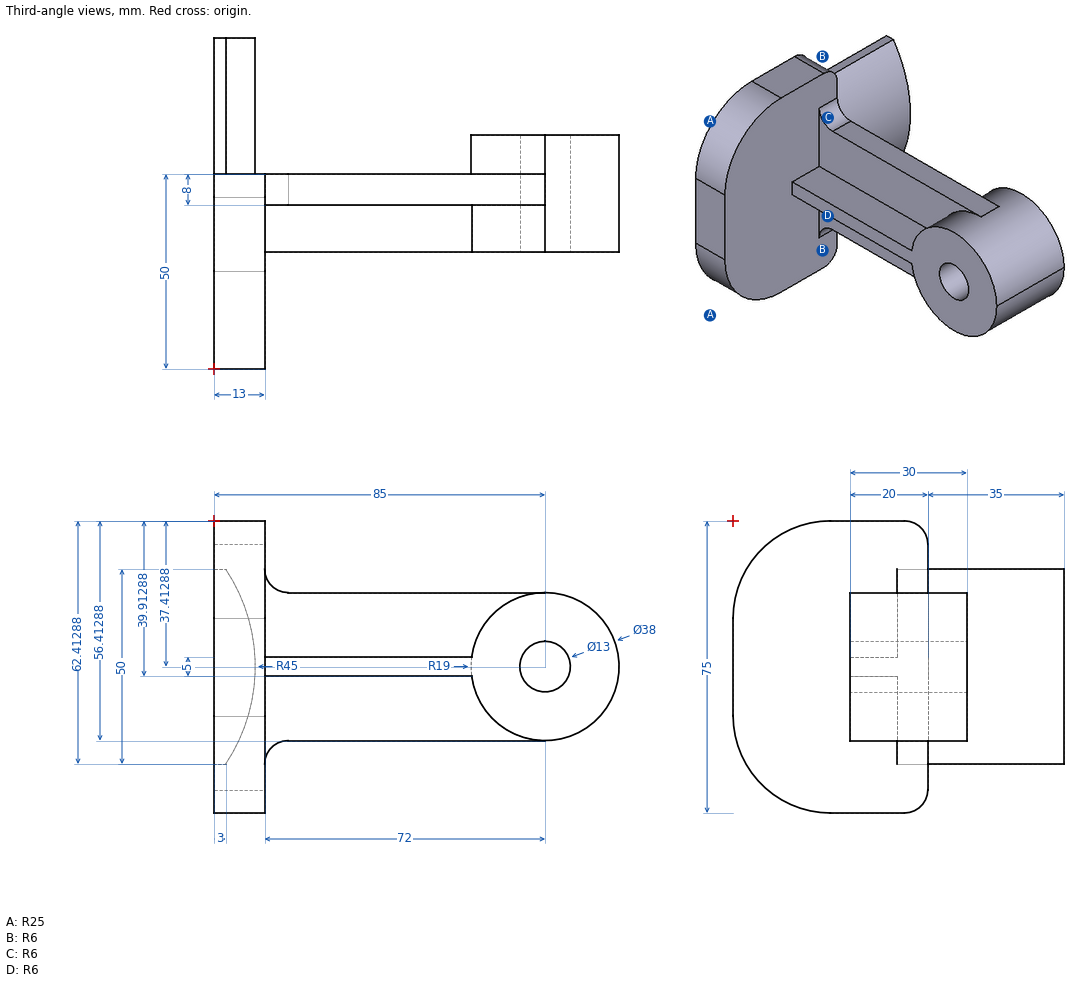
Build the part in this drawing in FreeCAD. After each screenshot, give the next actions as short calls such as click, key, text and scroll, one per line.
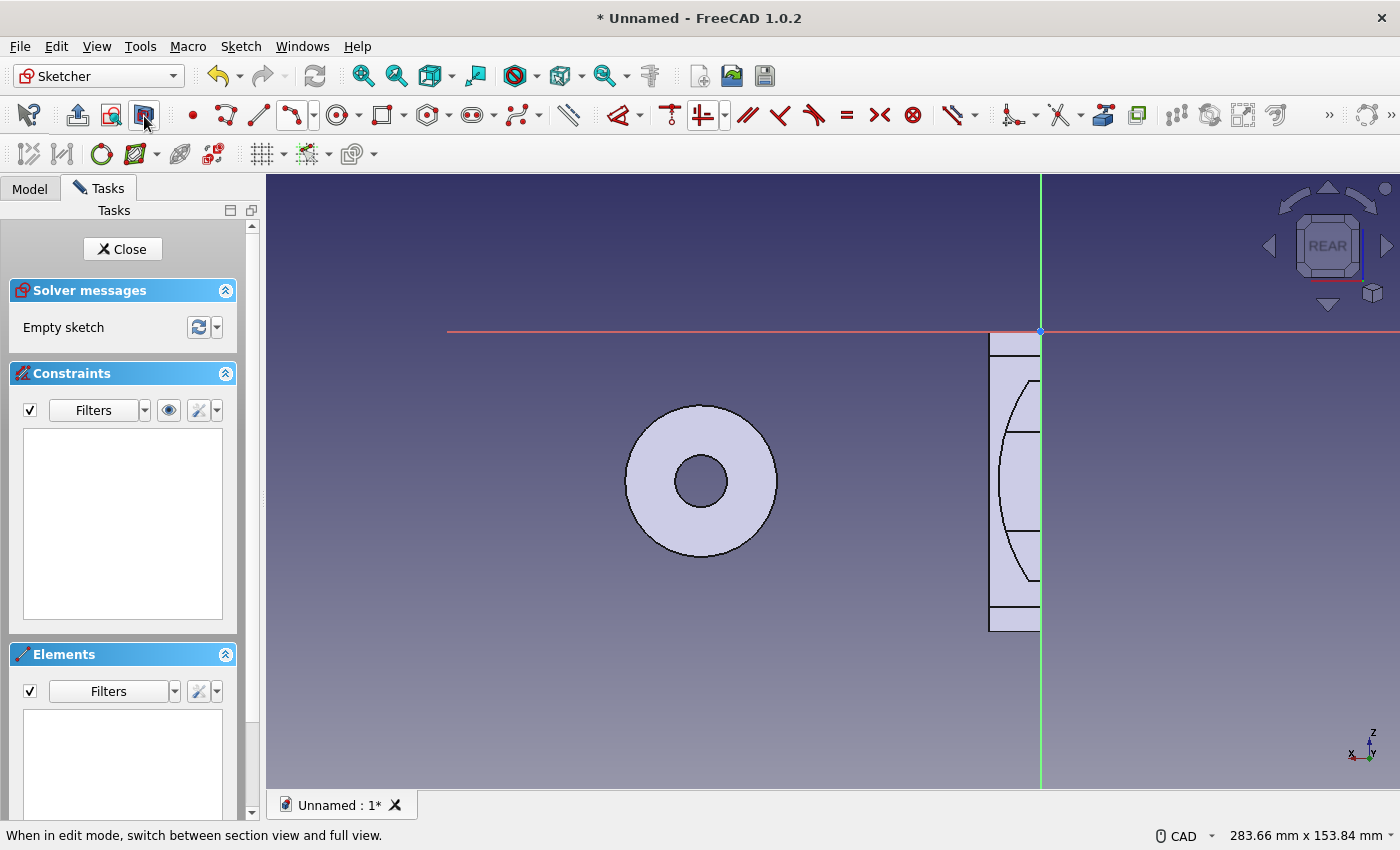
scroll(1000, 399, up, 3)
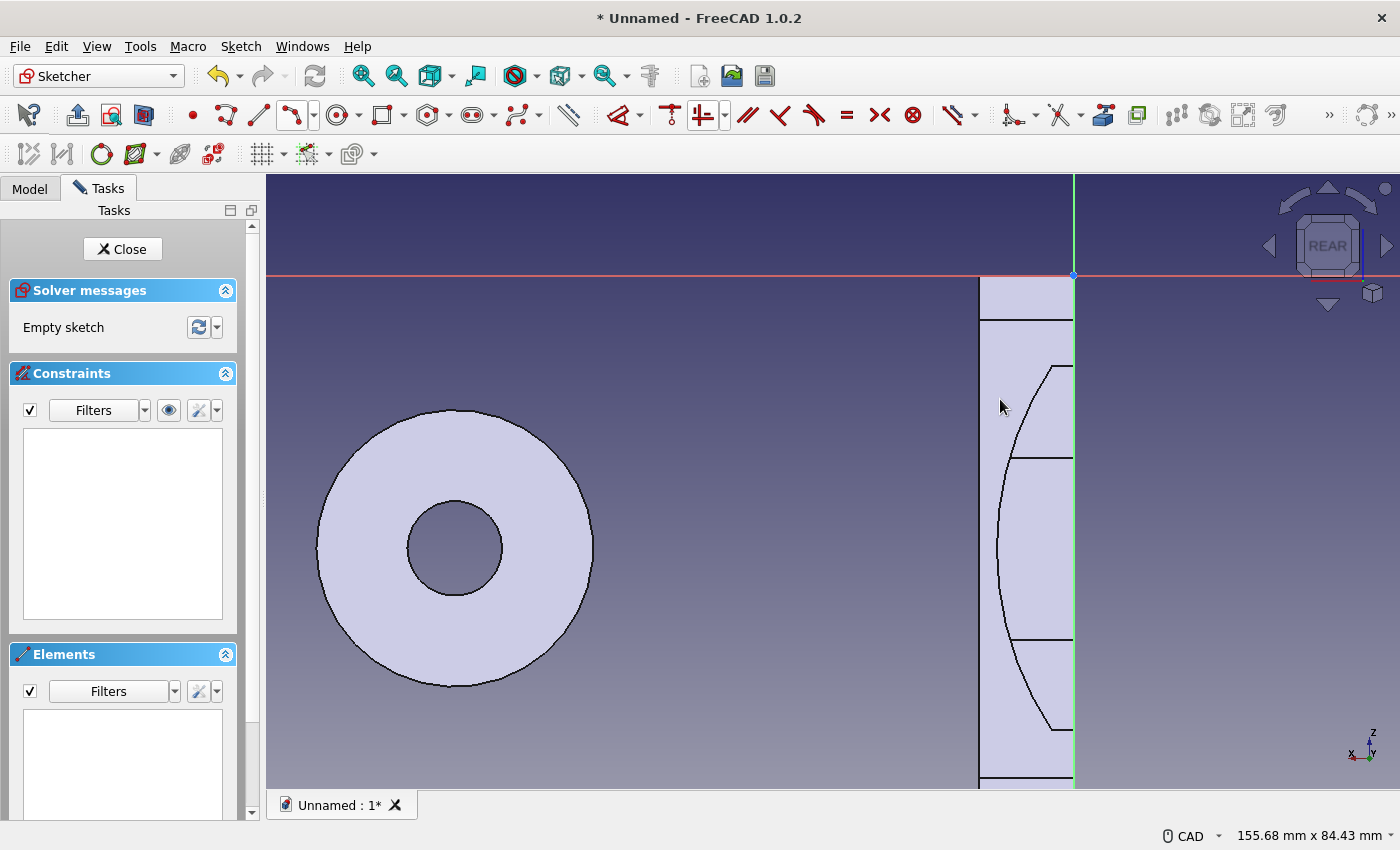
click(226, 116)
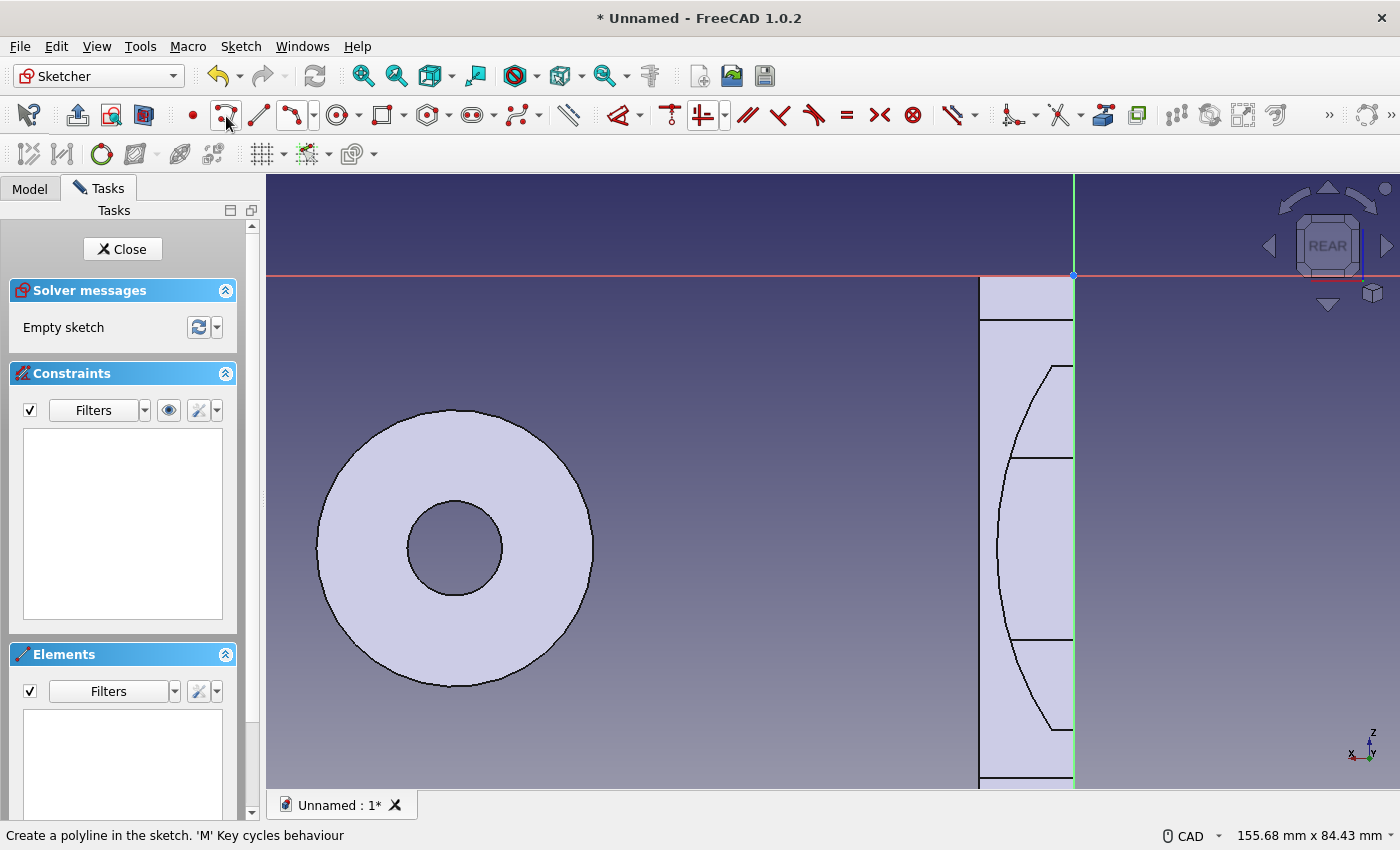
click(455, 687)
click(979, 687)
click(979, 410)
click(455, 410)
right_click(455, 410)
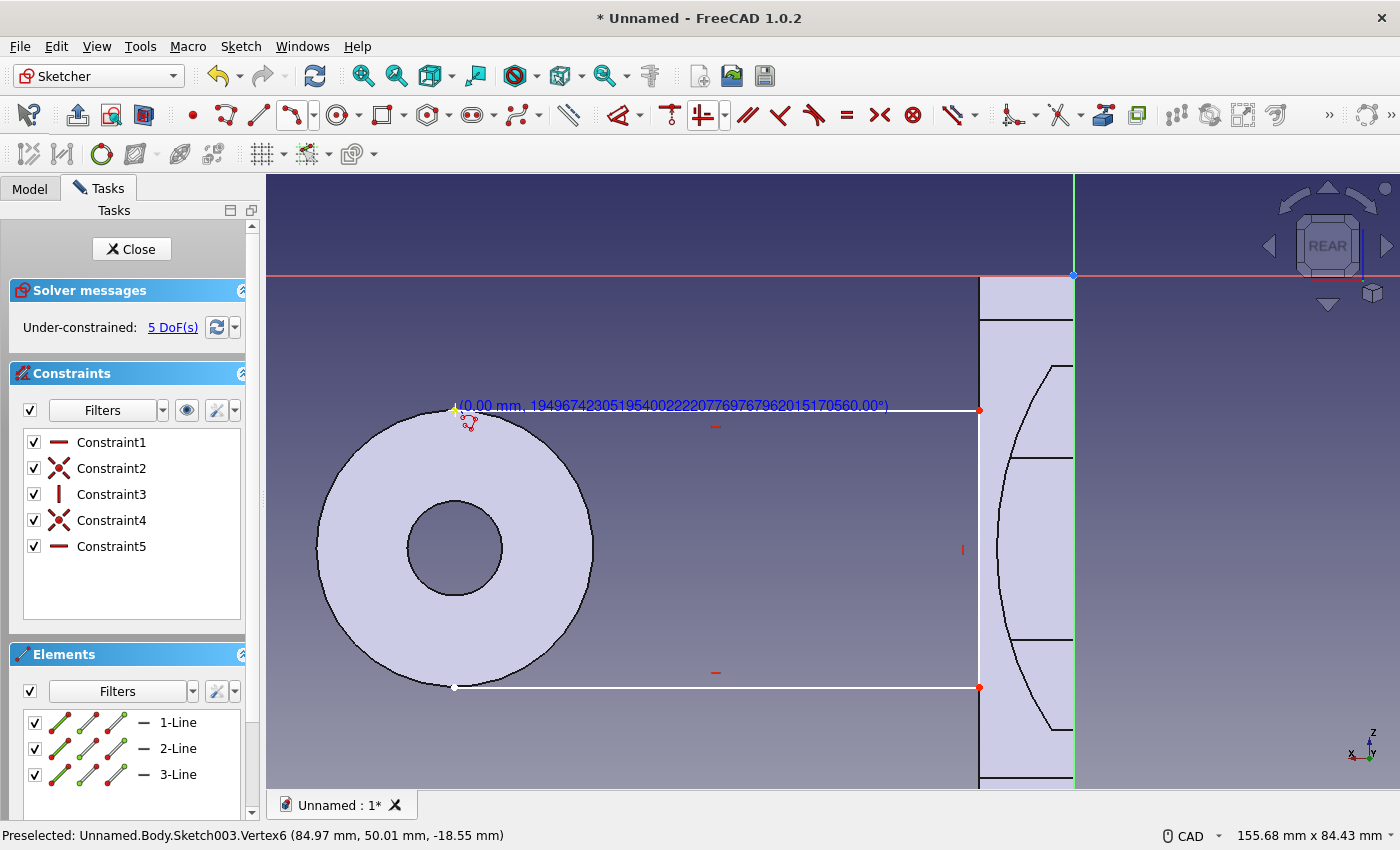
click(292, 116)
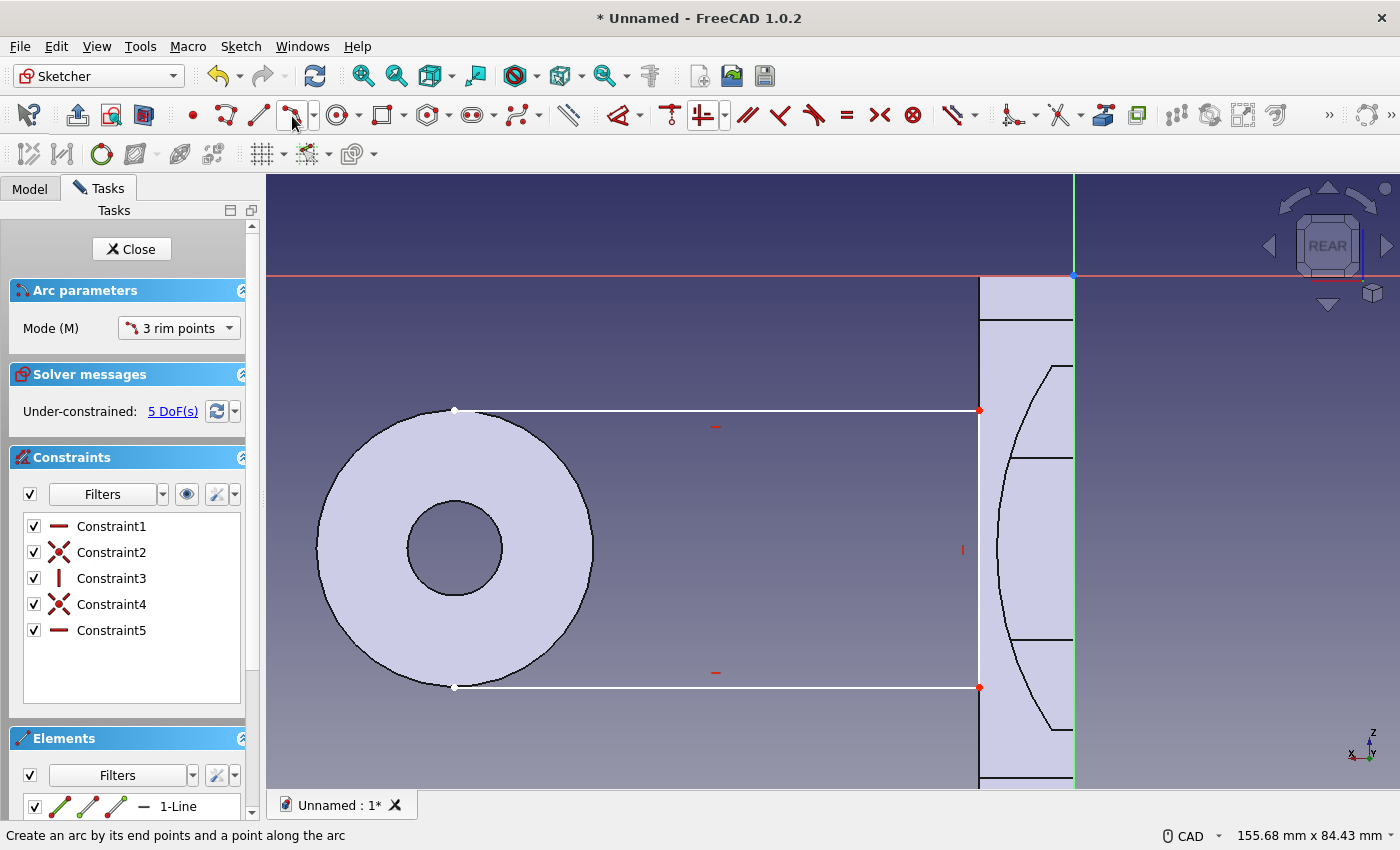
click(455, 411)
click(455, 688)
click(593, 548)
key(Escape)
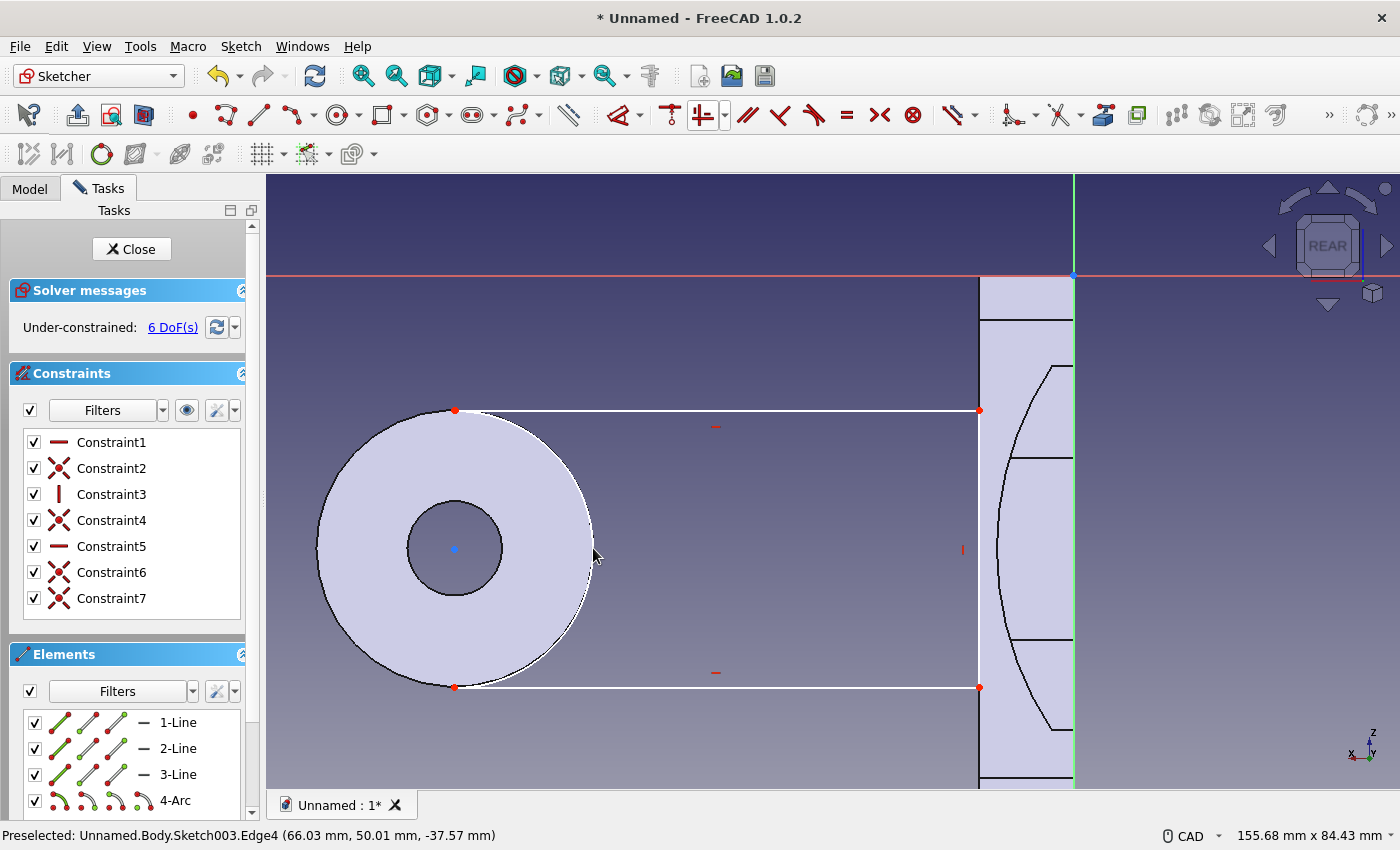
click(612, 688)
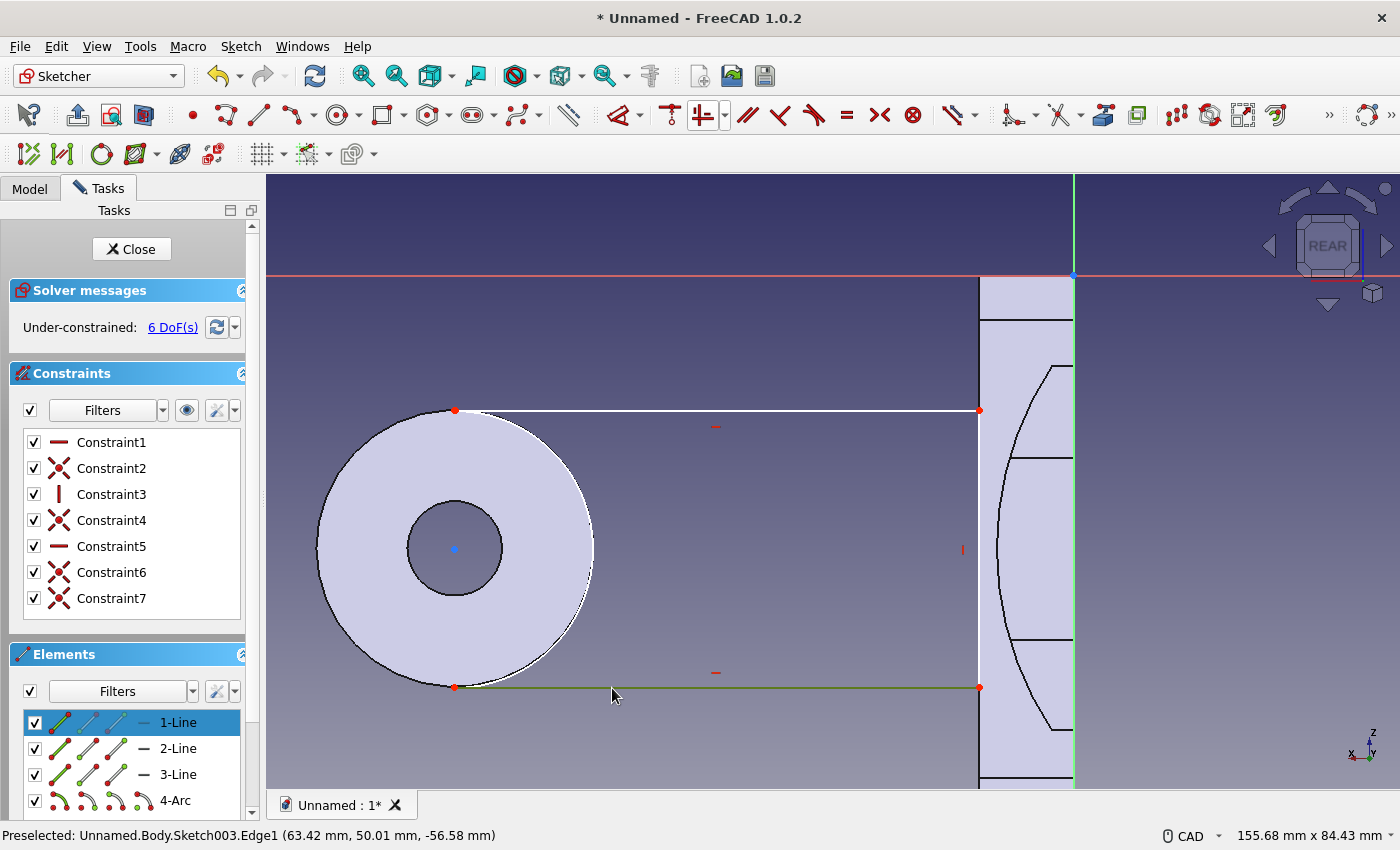
click(567, 631)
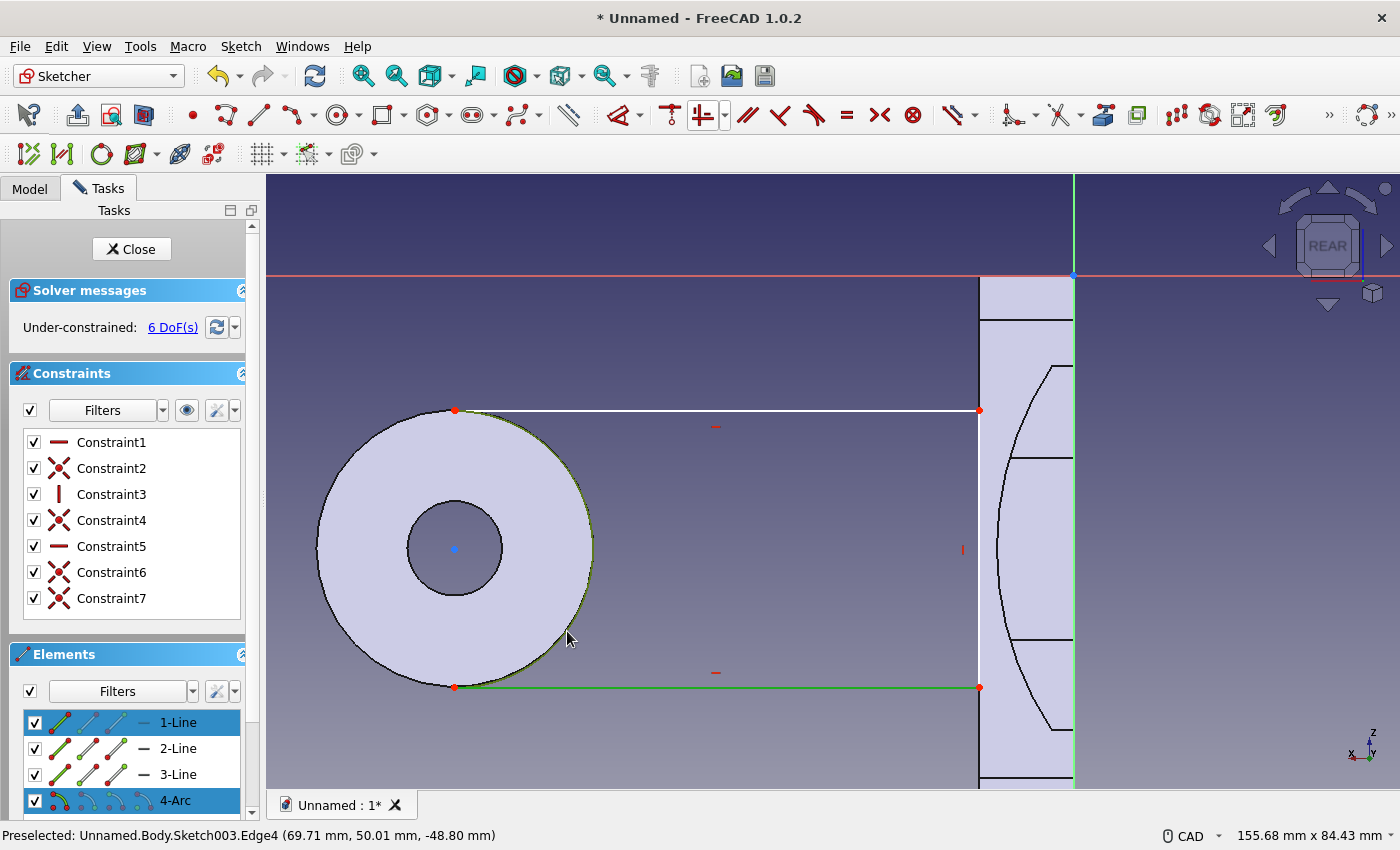
click(814, 116)